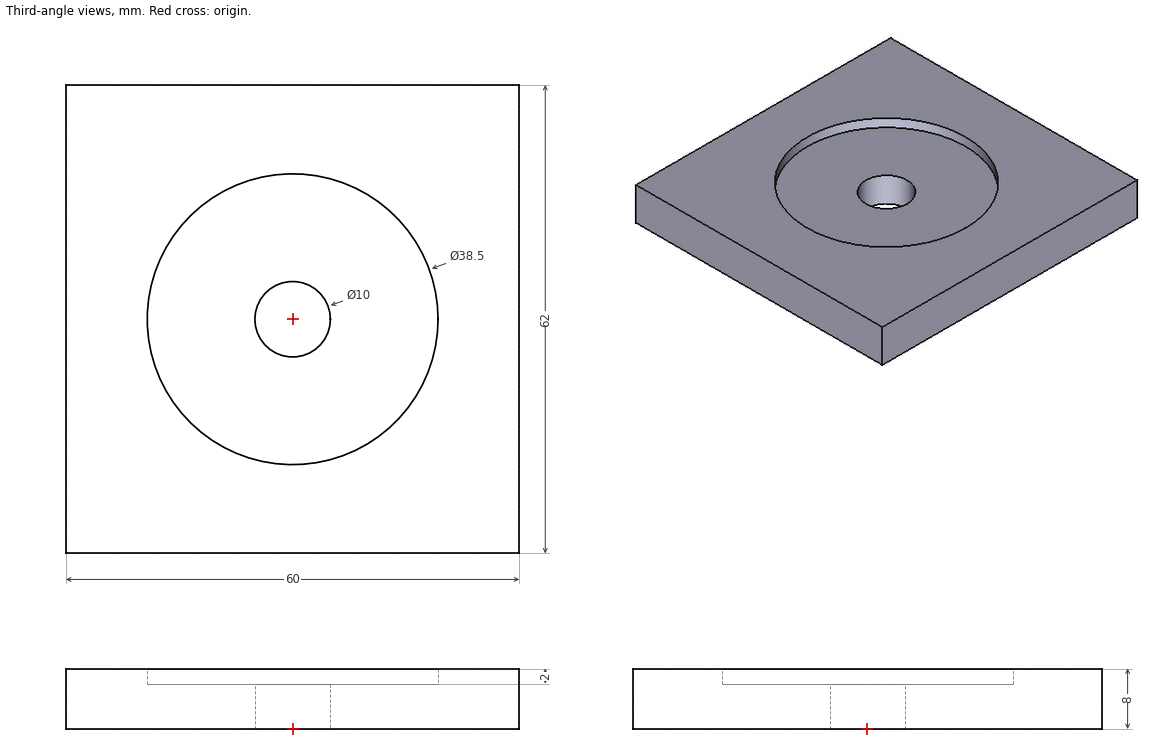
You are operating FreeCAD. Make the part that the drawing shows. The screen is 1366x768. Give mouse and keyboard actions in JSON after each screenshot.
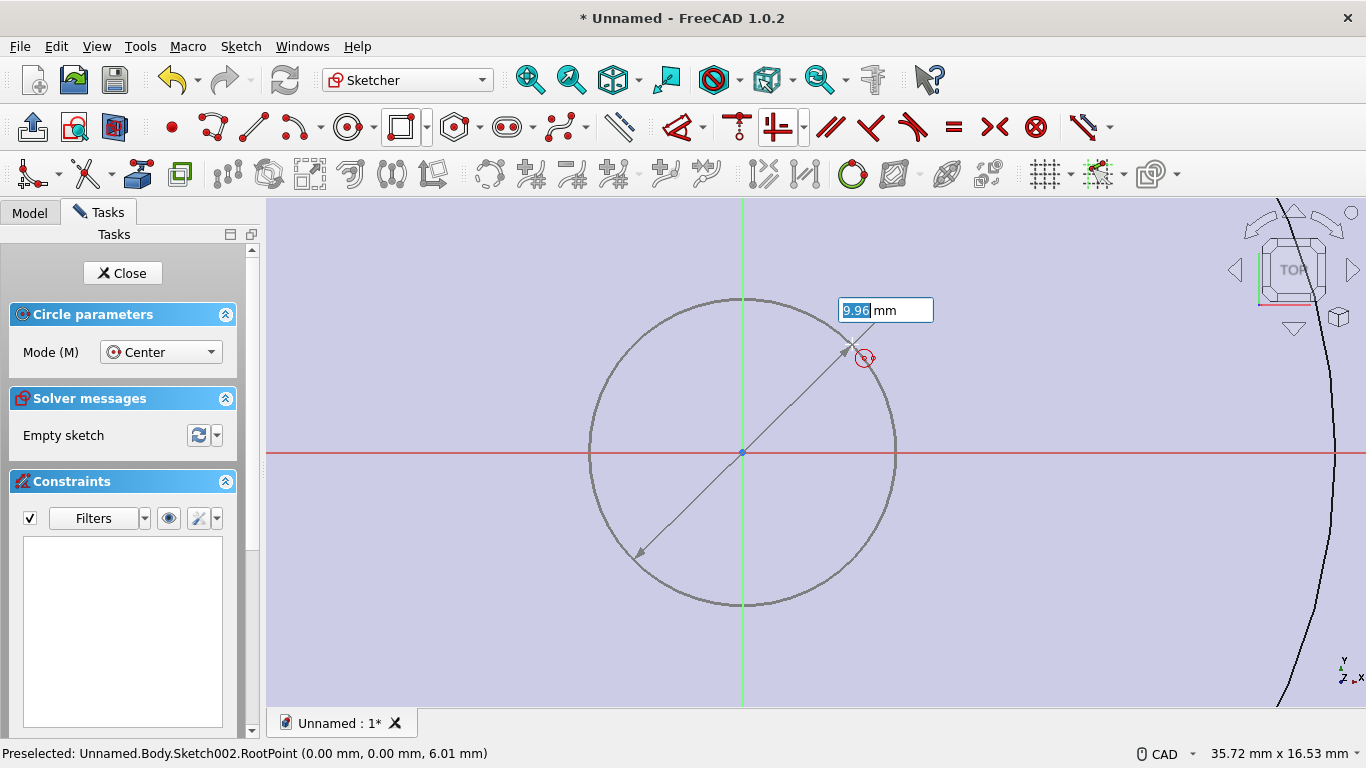
{"action": "type", "text": "10"}
{"action": "key", "text": "Return"}
{"action": "key", "text": "Escape"}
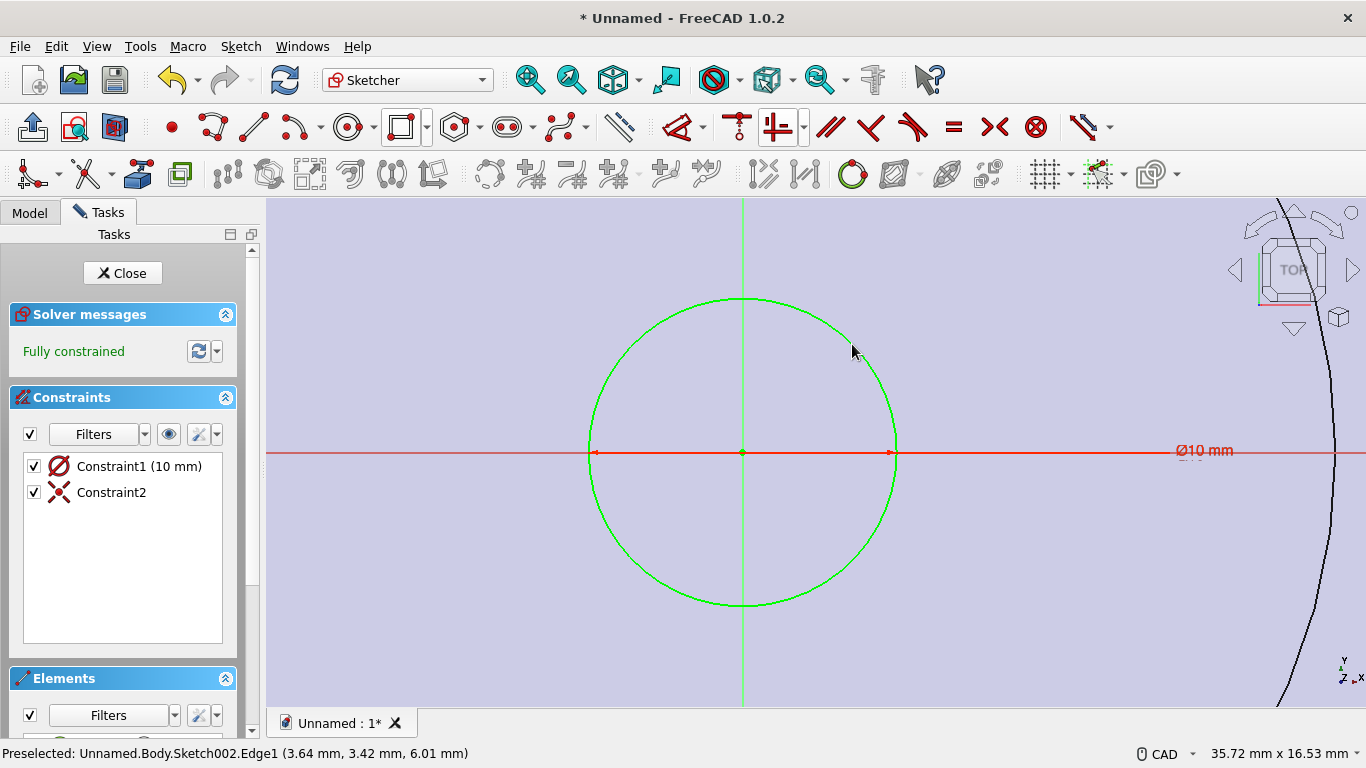
{"action": "left_click", "coordinate": [123, 273]}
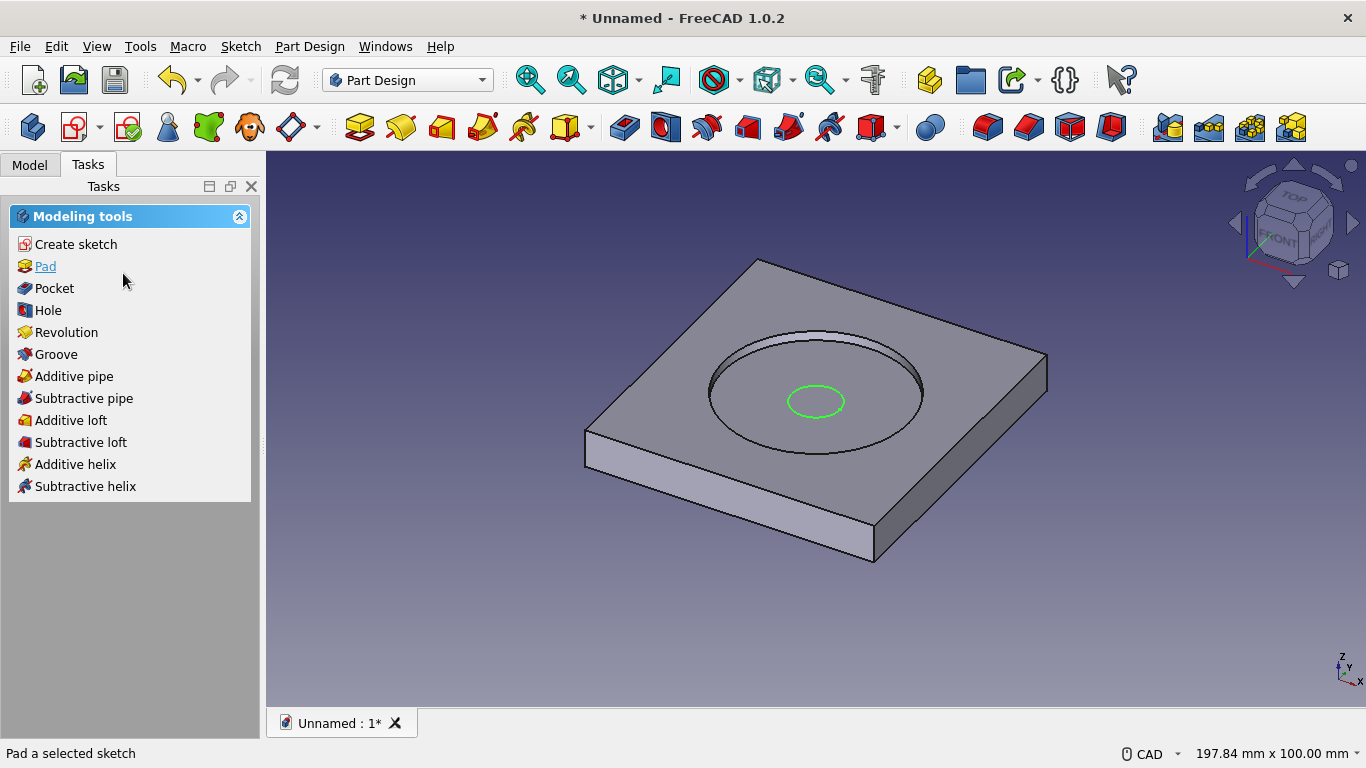
{"action": "left_click", "coordinate": [625, 128]}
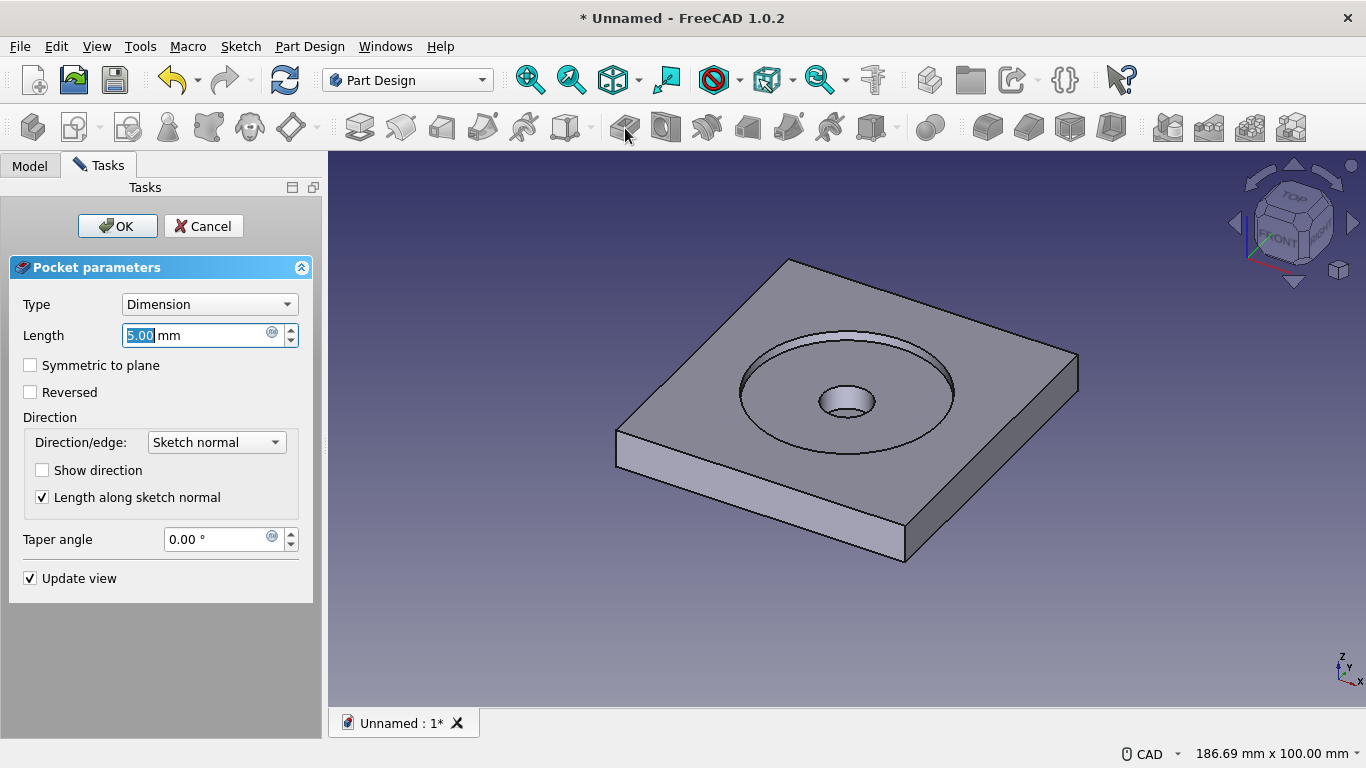
{"action": "left_click", "coordinate": [210, 304]}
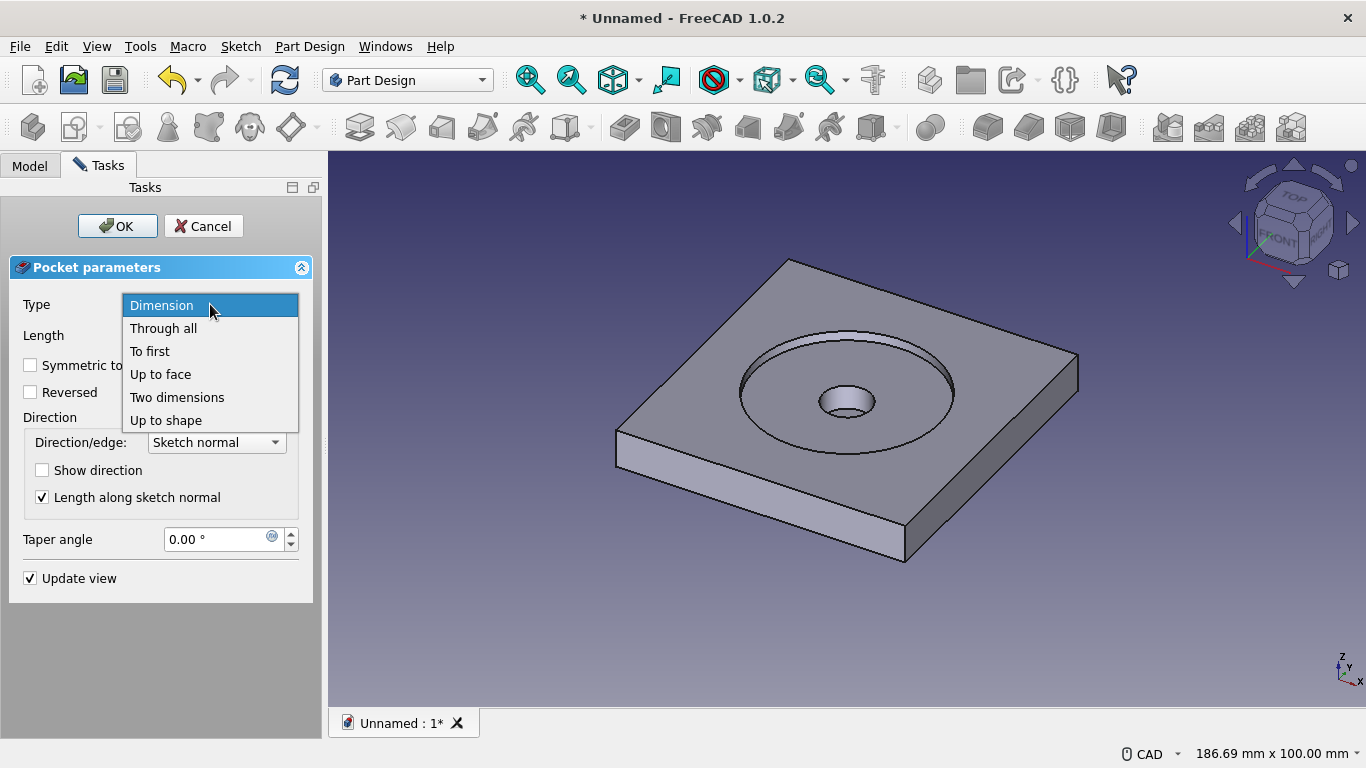
{"action": "left_click", "coordinate": [208, 328]}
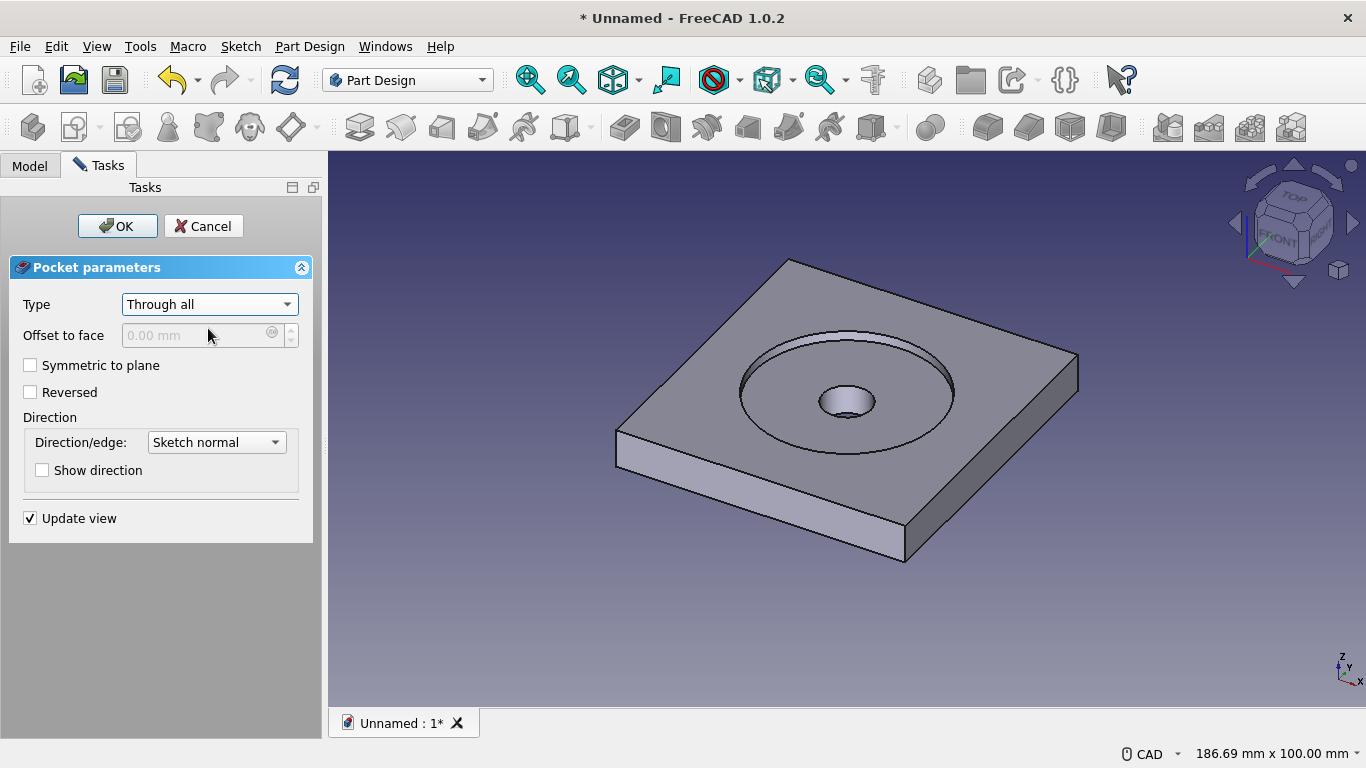
{"action": "left_click", "coordinate": [118, 226]}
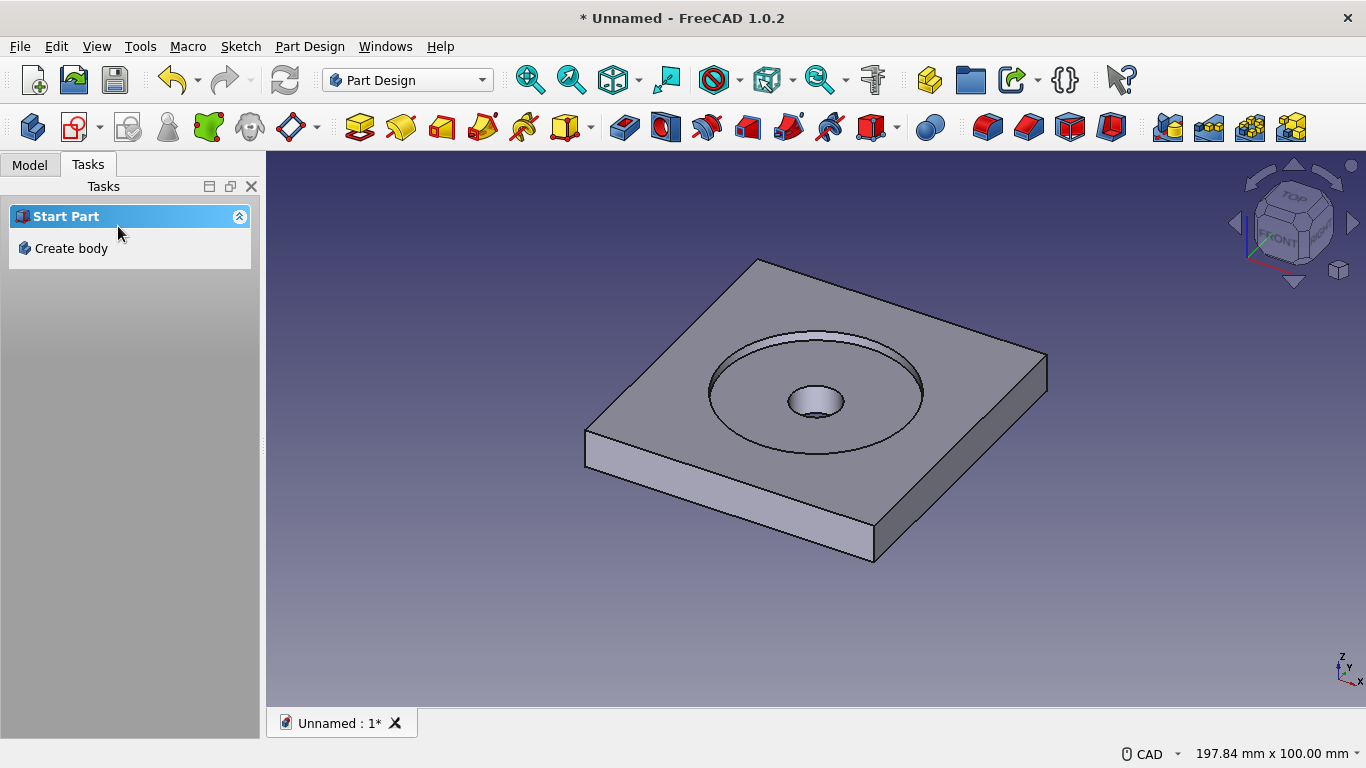
{"action": "key", "text": "0"}